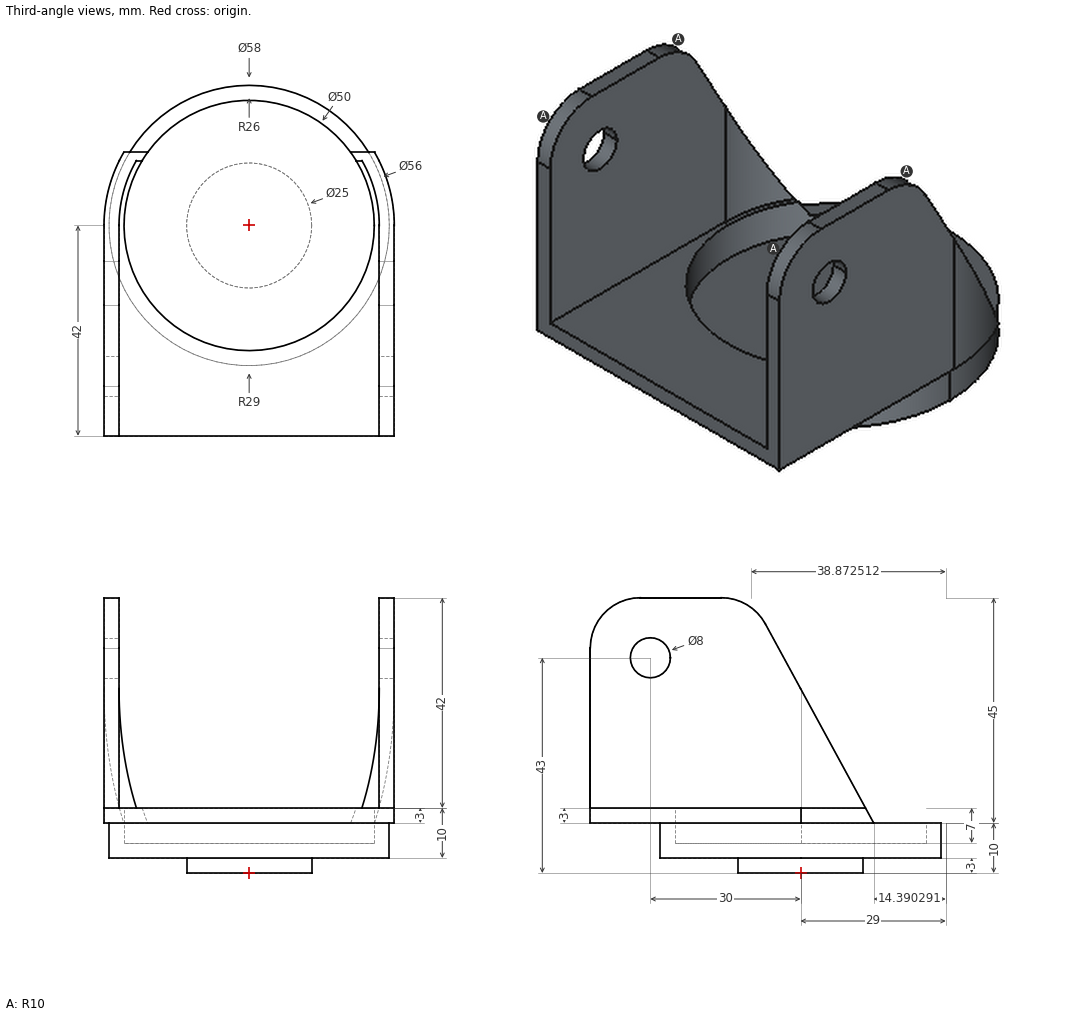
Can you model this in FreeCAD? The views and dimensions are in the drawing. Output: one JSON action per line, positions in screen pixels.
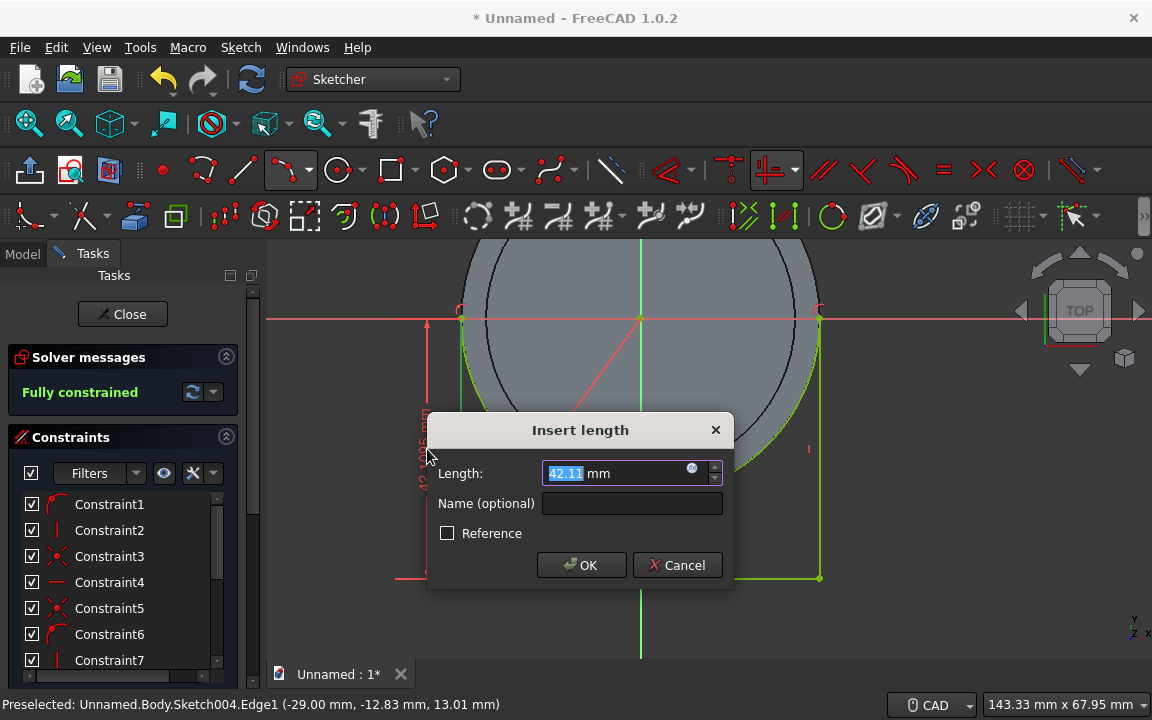
{"action": "type", "text": "42"}
{"action": "key", "text": "Return"}
{"action": "key", "text": "Escape"}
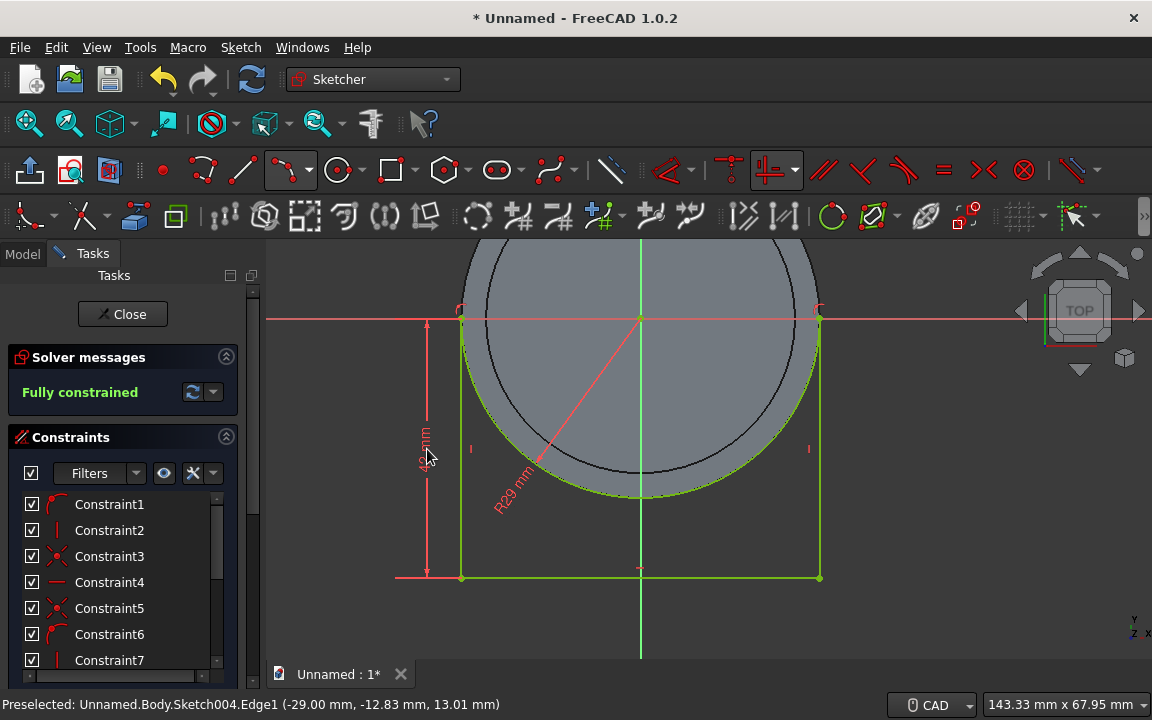
{"action": "left_click", "coordinate": [123, 314]}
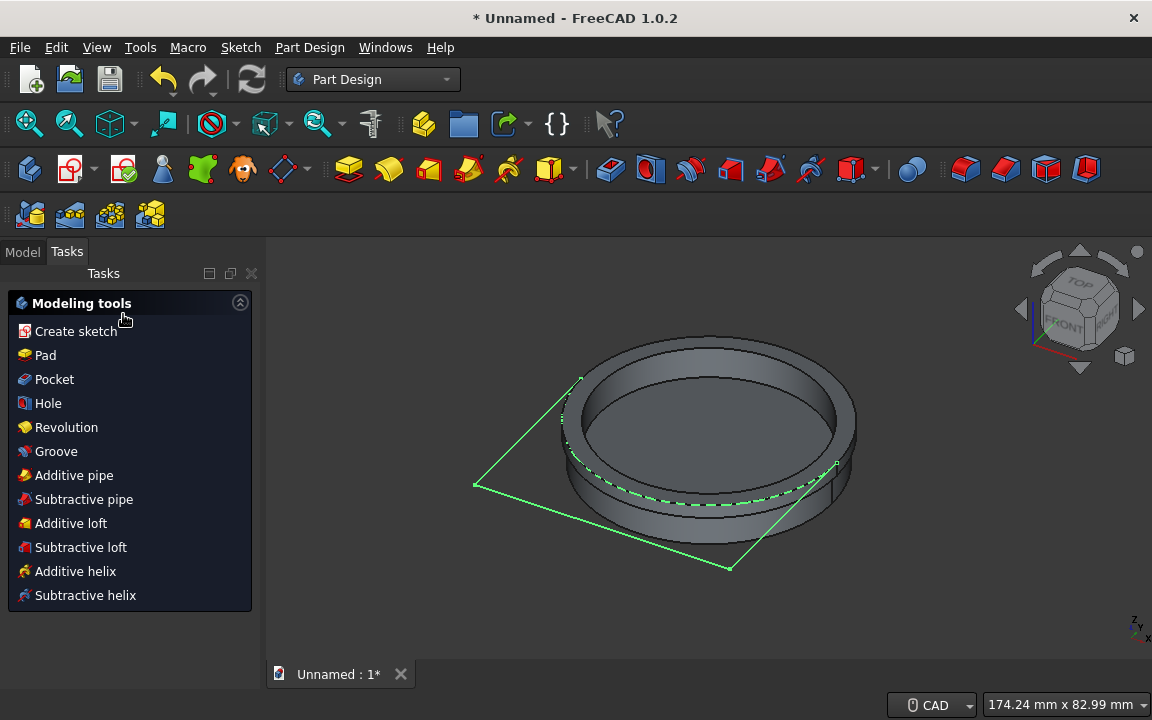
{"action": "left_click", "coordinate": [350, 170]}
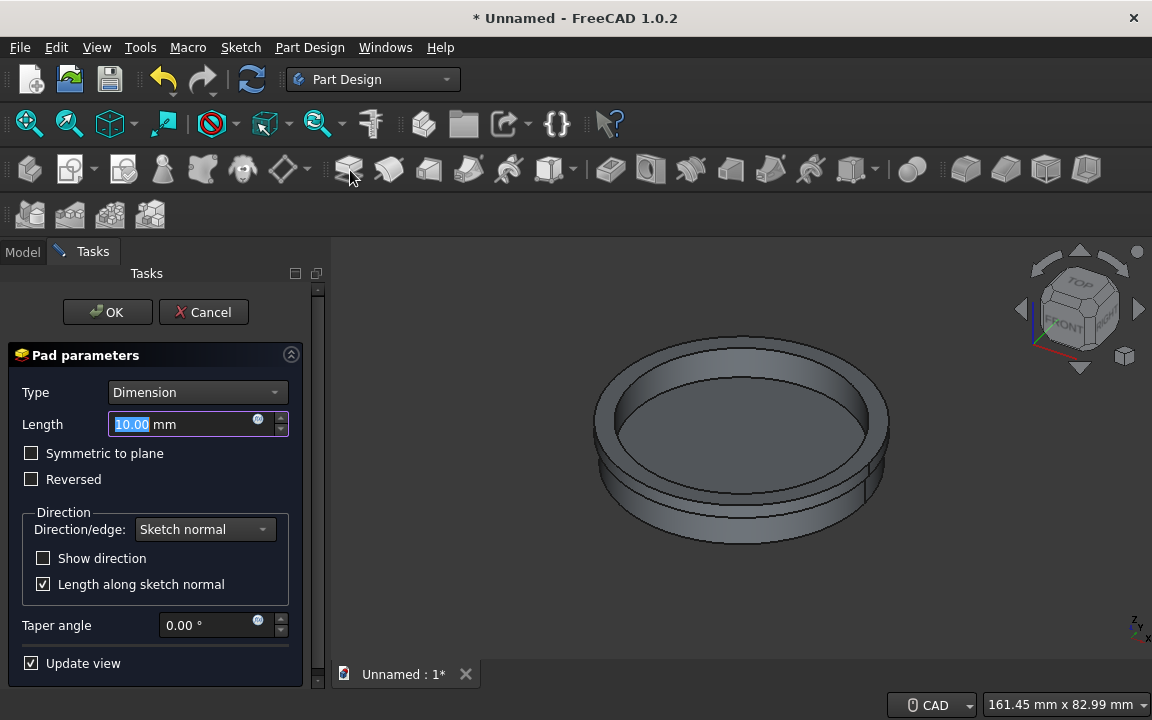
{"action": "type", "text": "3"}
{"action": "key", "text": "Tab"}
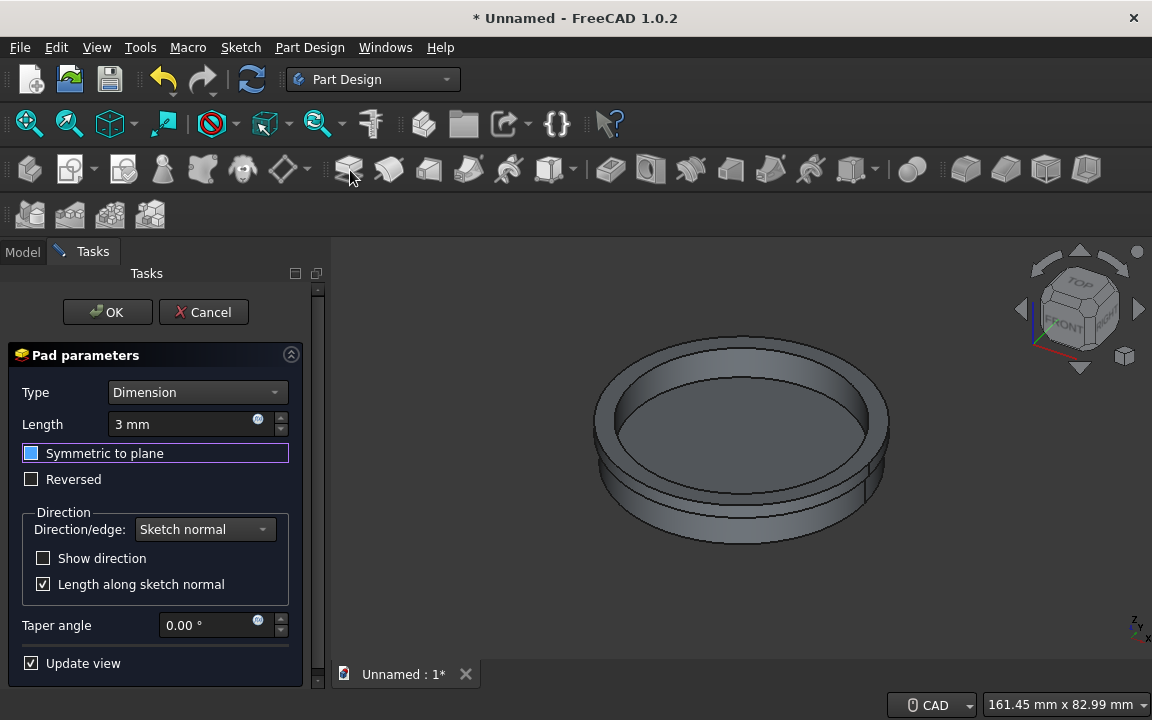
{"action": "left_click", "coordinate": [30, 479]}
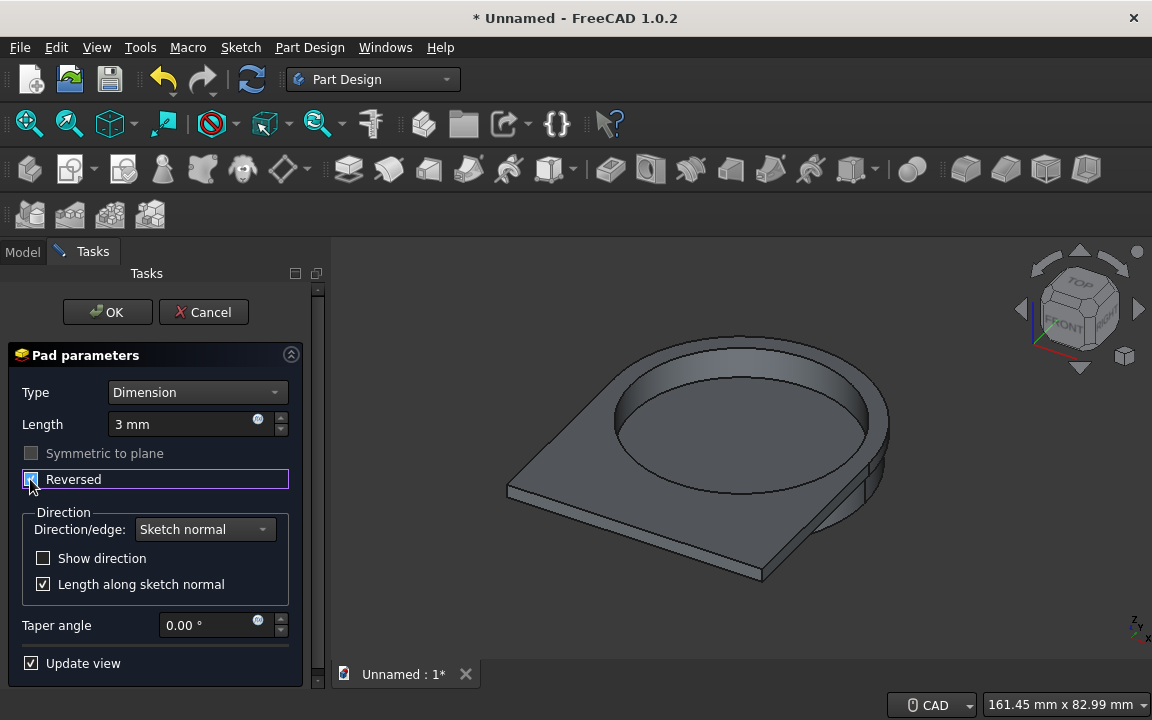
{"action": "left_click", "coordinate": [108, 312]}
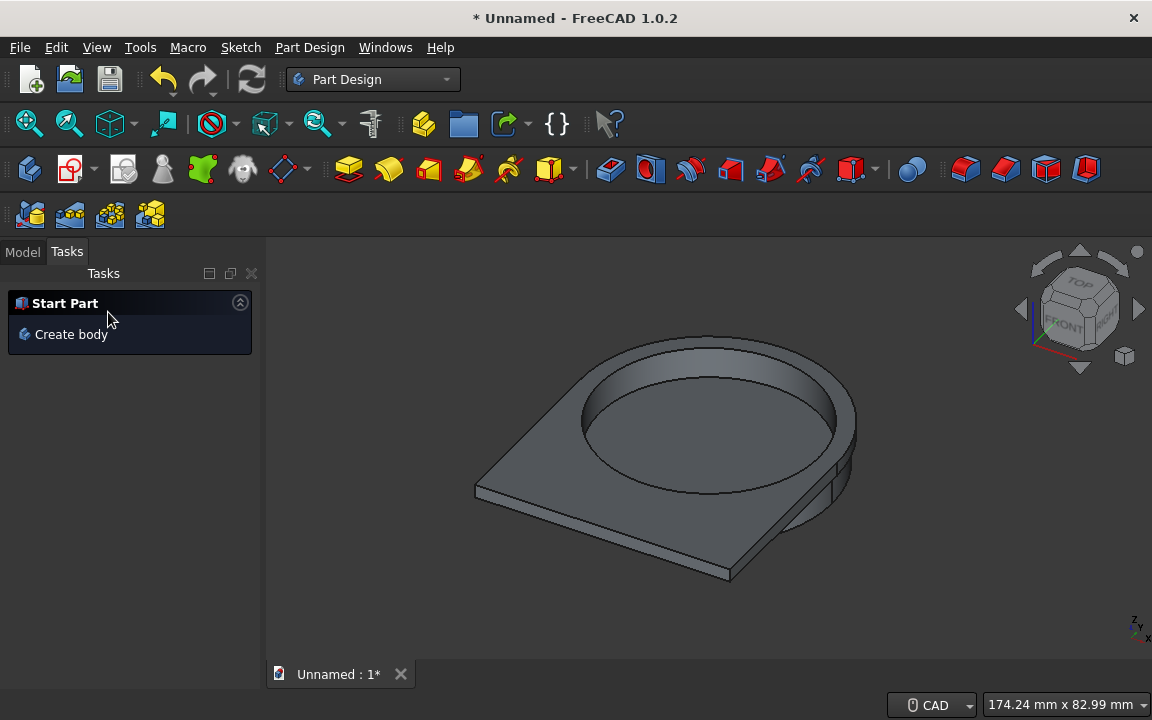
{"action": "left_click", "coordinate": [23, 251]}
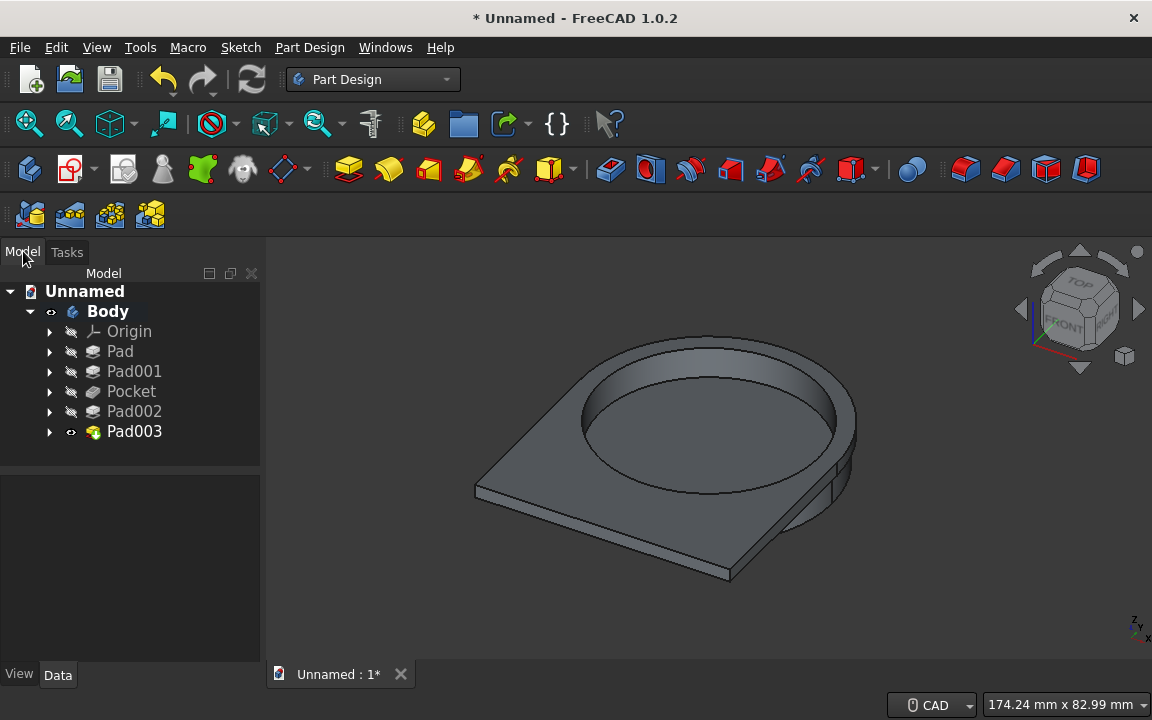
{"action": "left_click", "coordinate": [50, 332]}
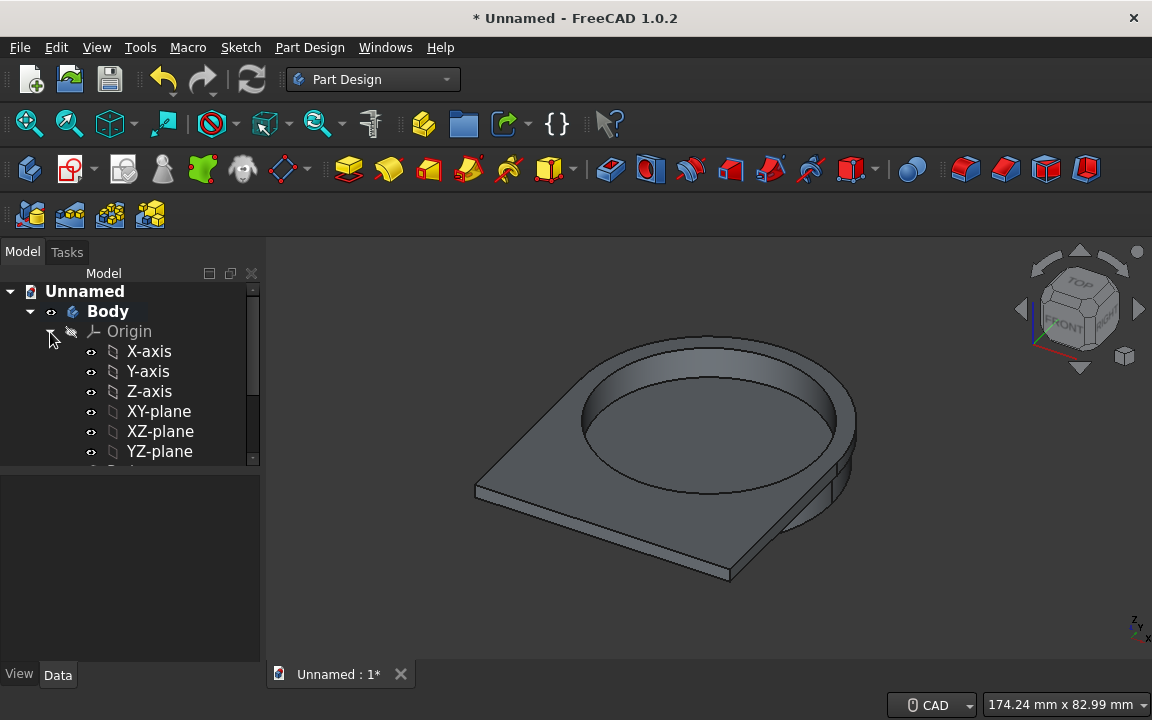
{"action": "left_click", "coordinate": [136, 412]}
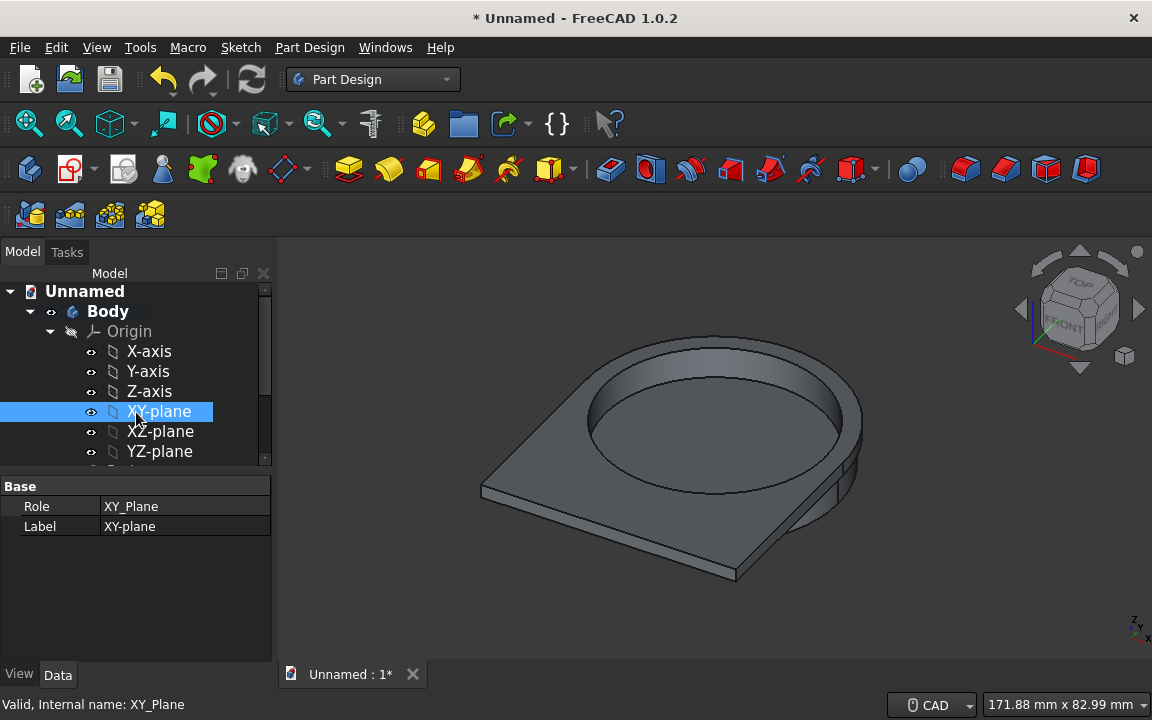
{"action": "left_click", "coordinate": [284, 170]}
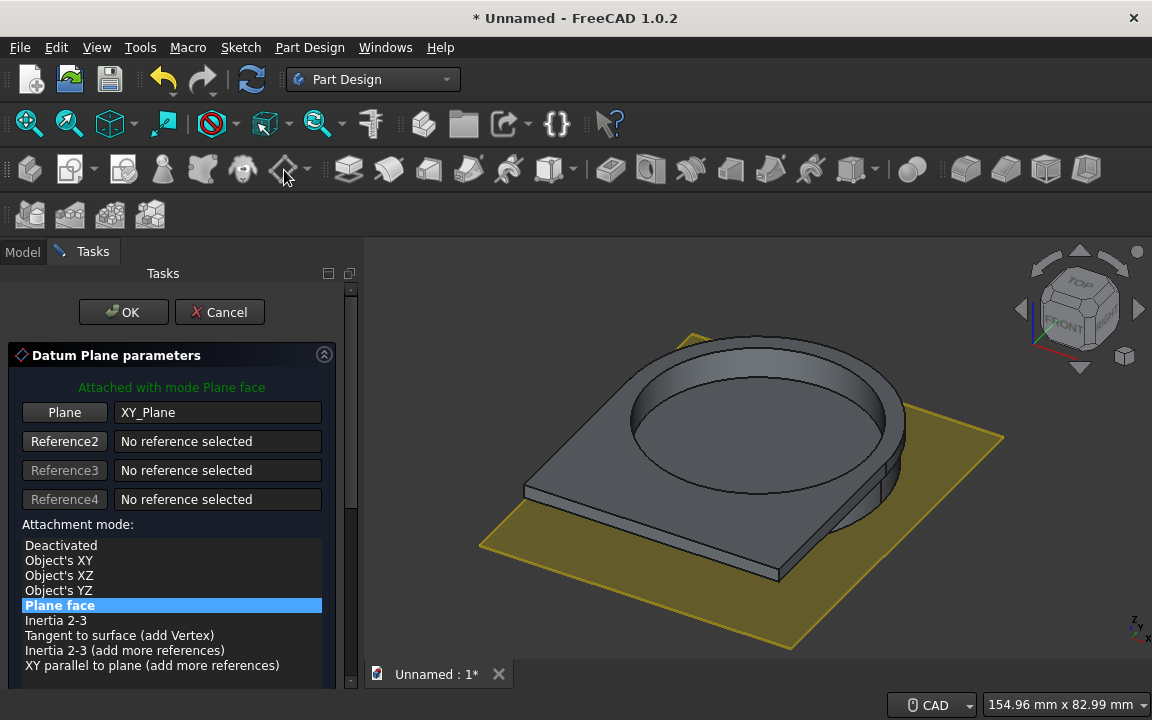
{"action": "scroll", "coordinate": [351, 486], "scroll_direction": "down", "scroll_amount": 4}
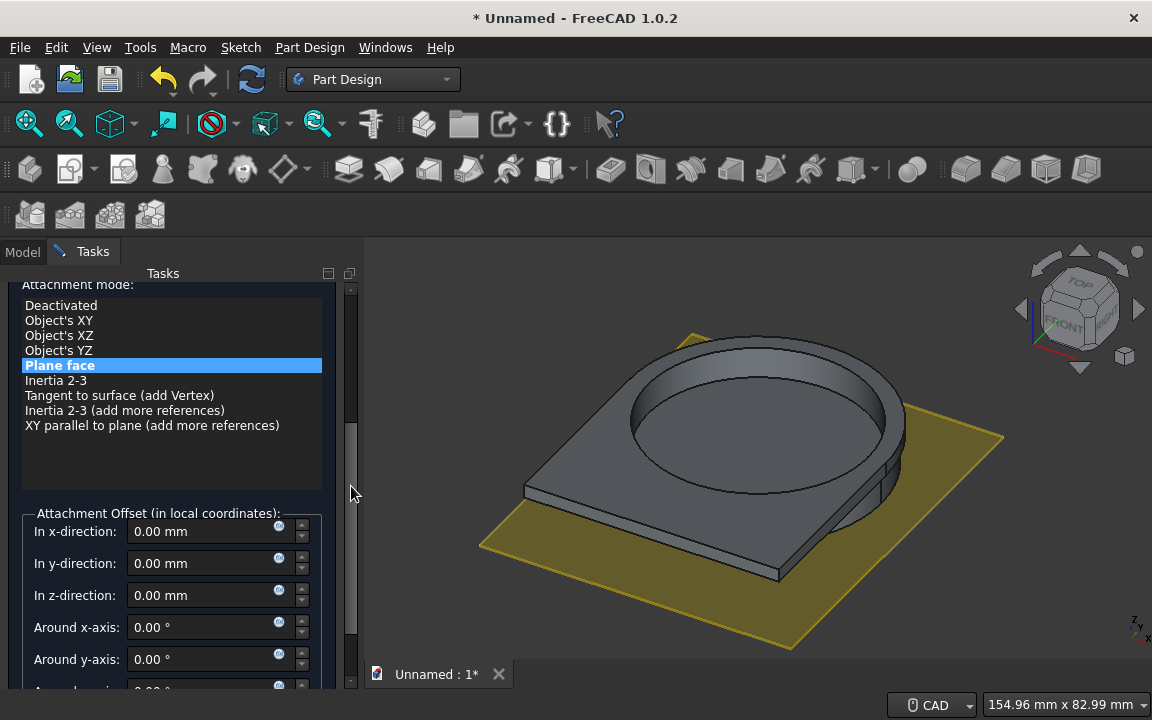
{"action": "triple_click", "coordinate": [210, 595]}